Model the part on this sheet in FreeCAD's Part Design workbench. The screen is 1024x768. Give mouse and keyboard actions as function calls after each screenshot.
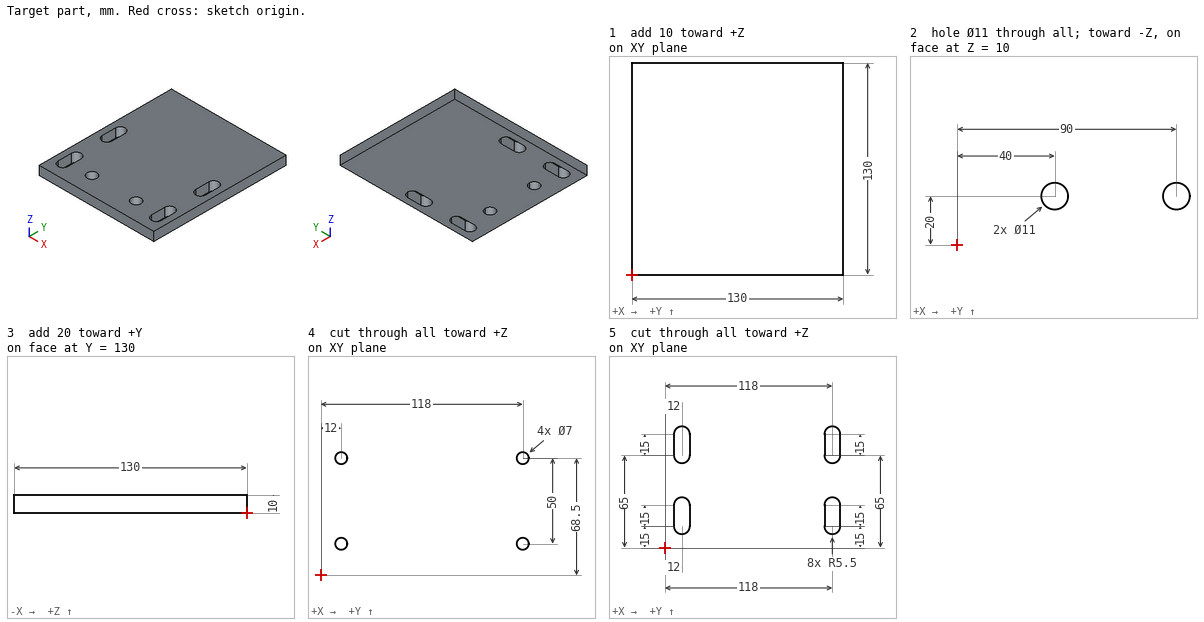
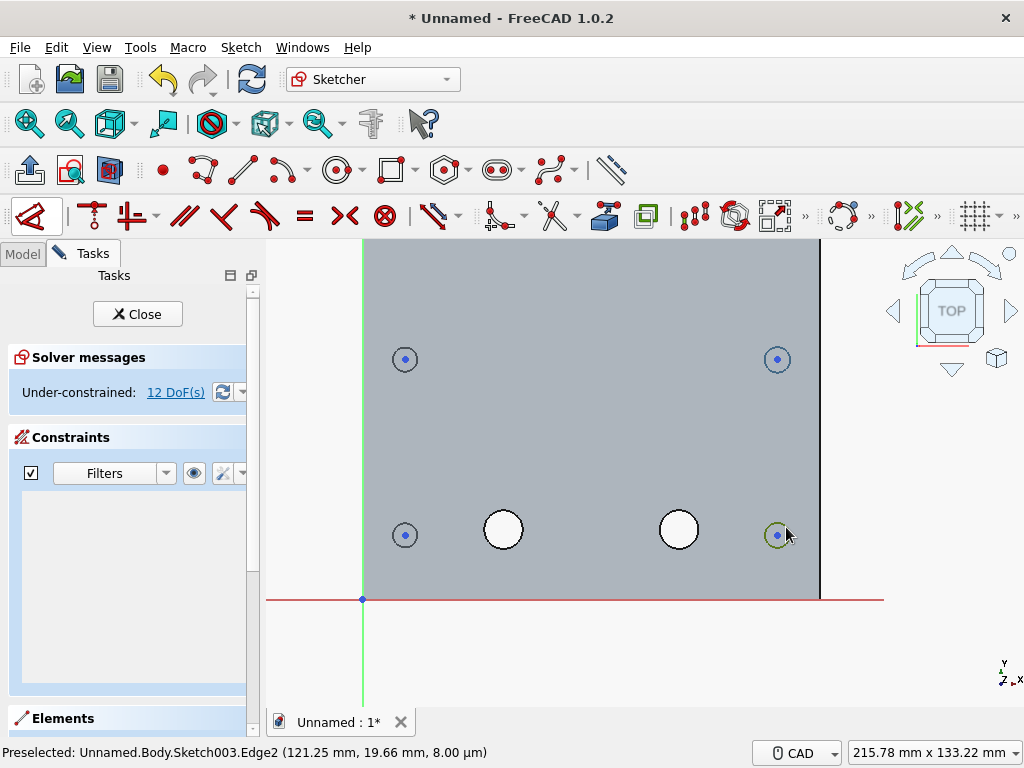
click(414, 351)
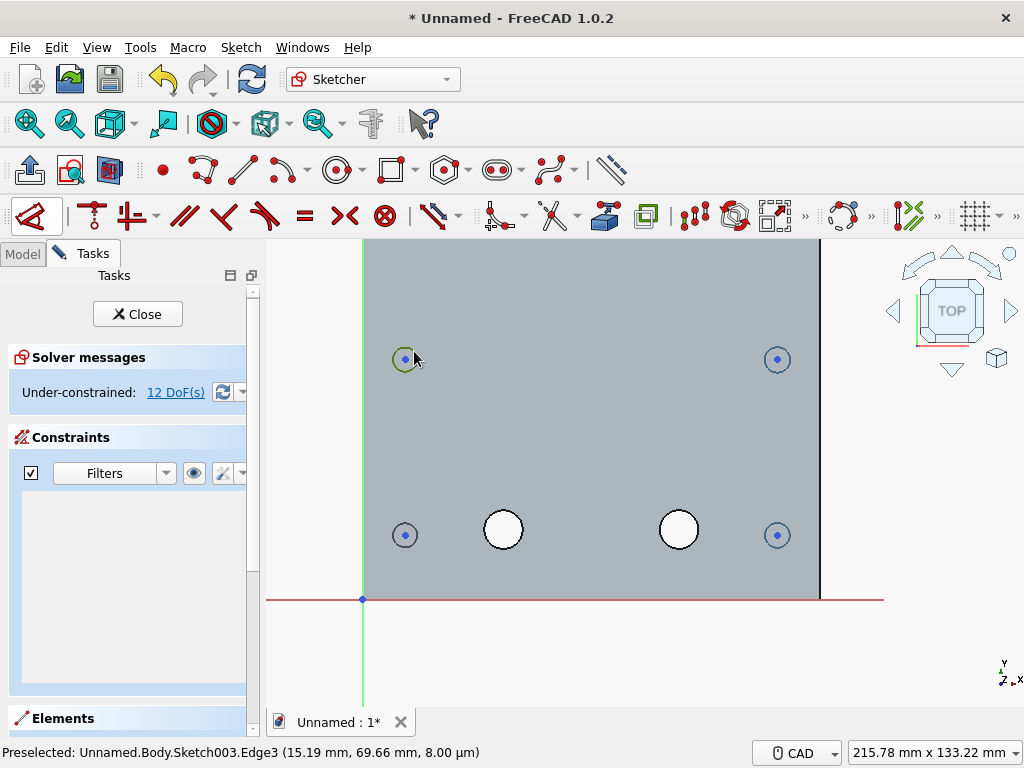
click(414, 527)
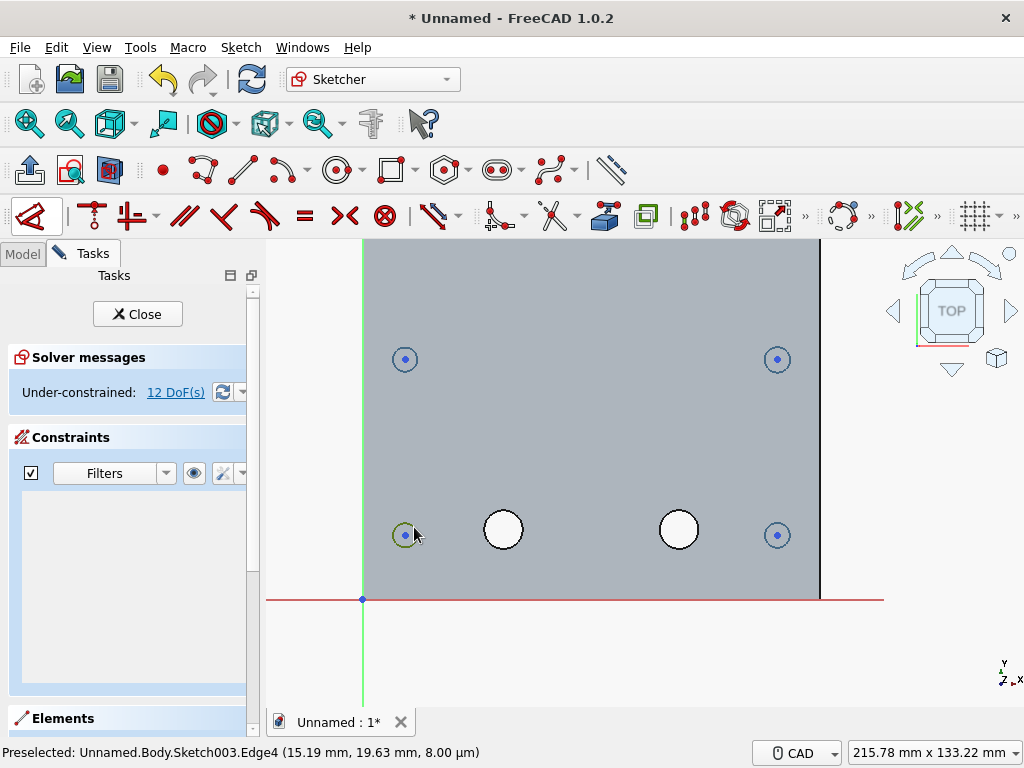
click(306, 216)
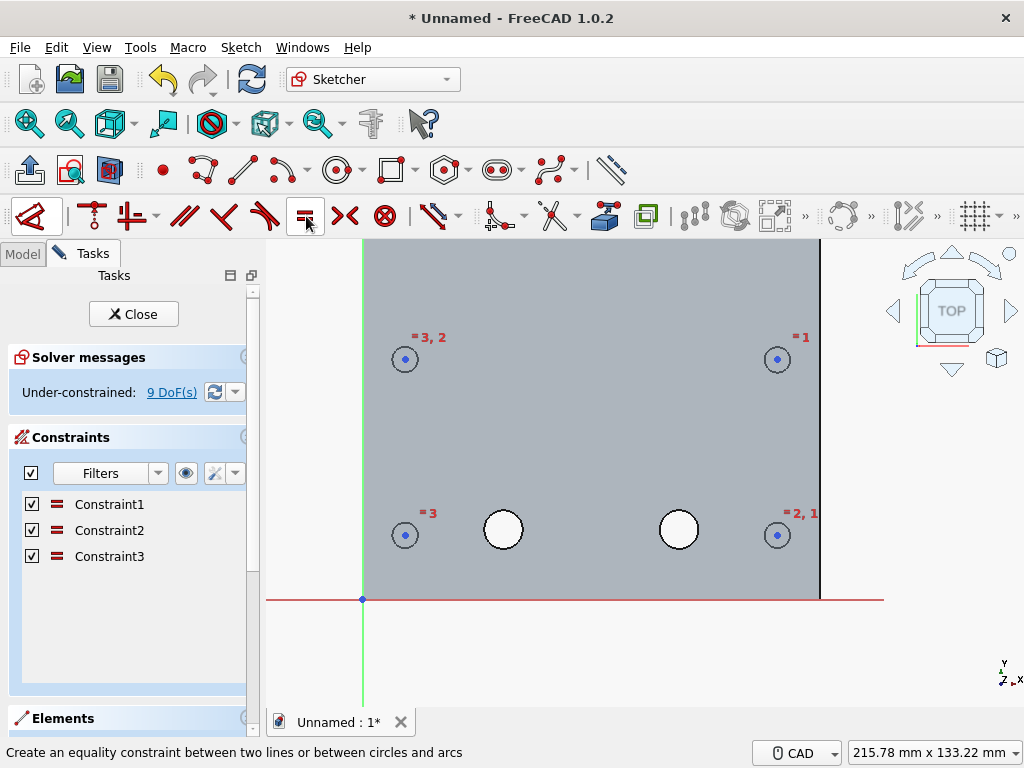
click(777, 360)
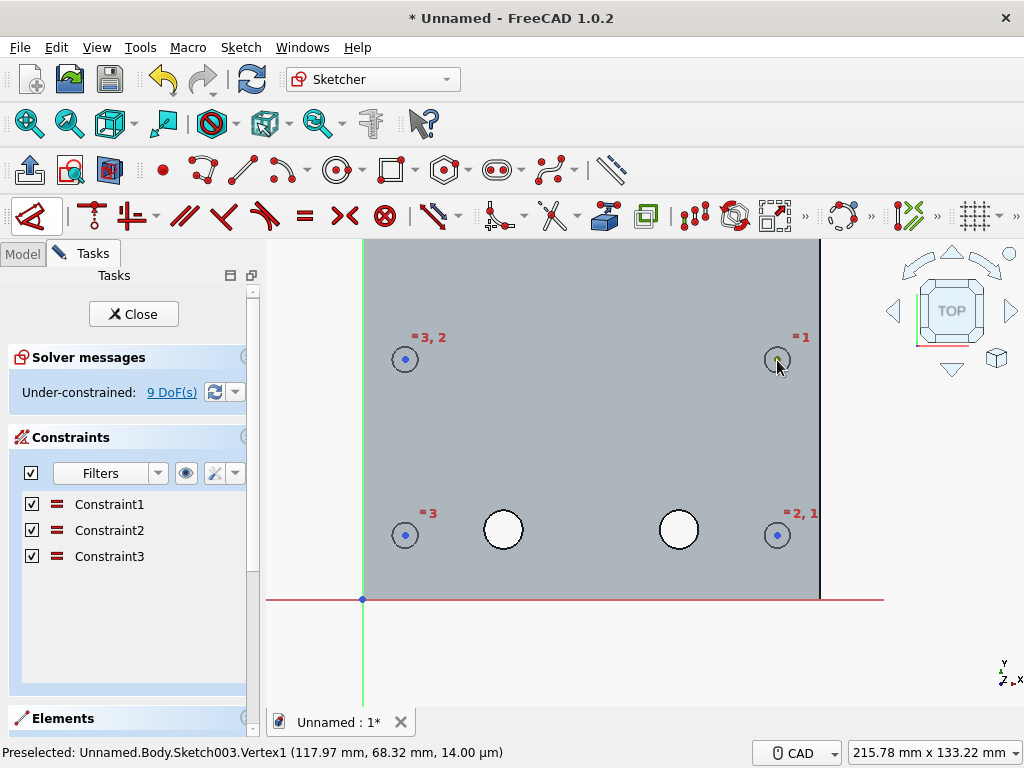
click(777, 535)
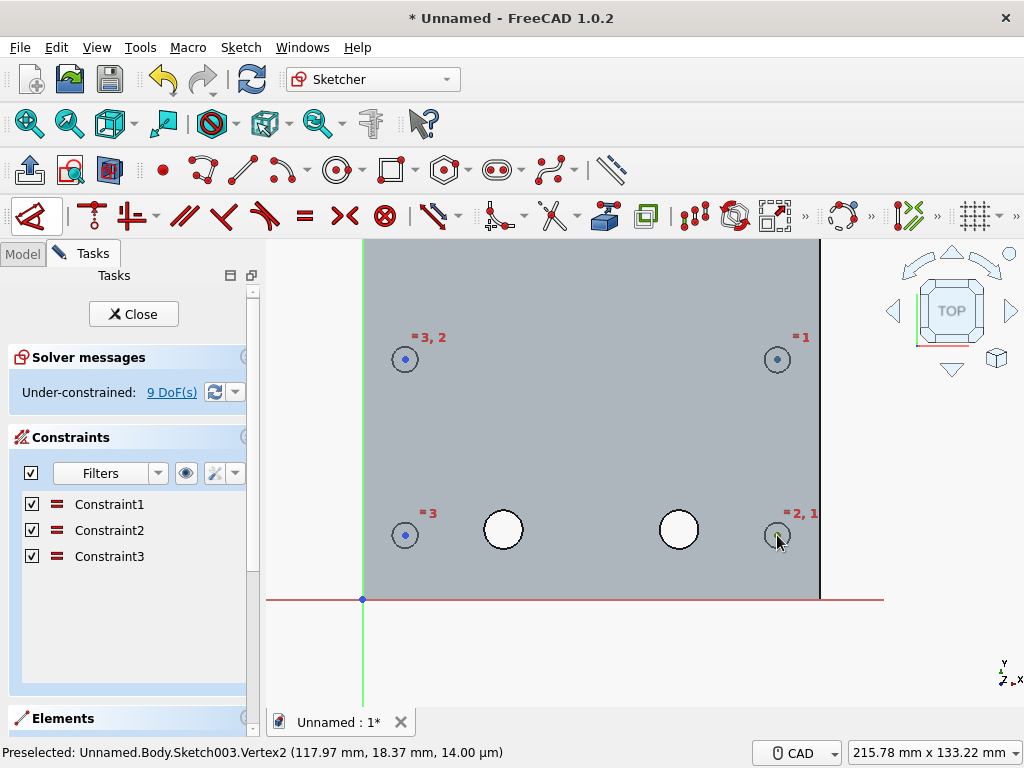
key(v)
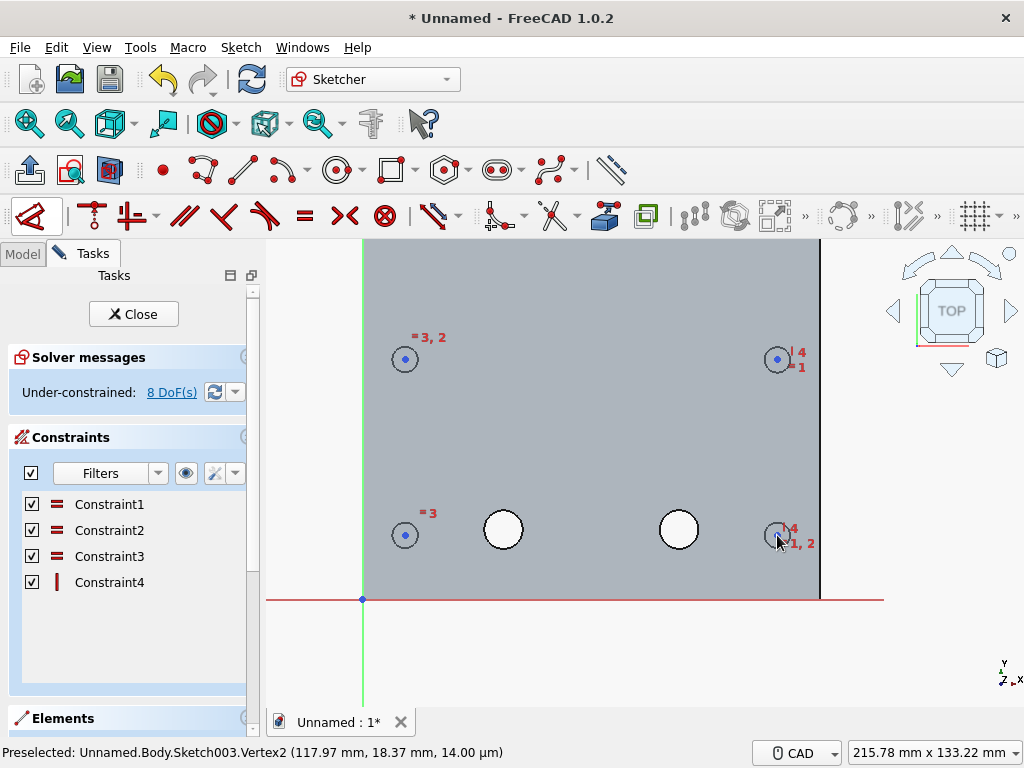
click(777, 360)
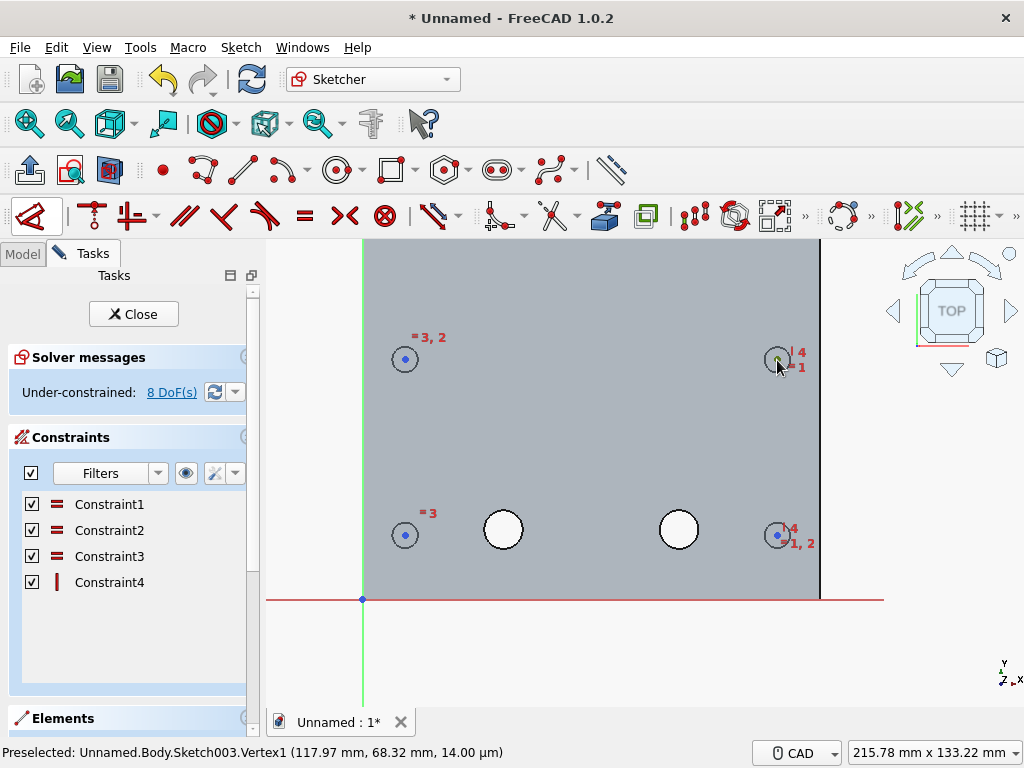
click(405, 360)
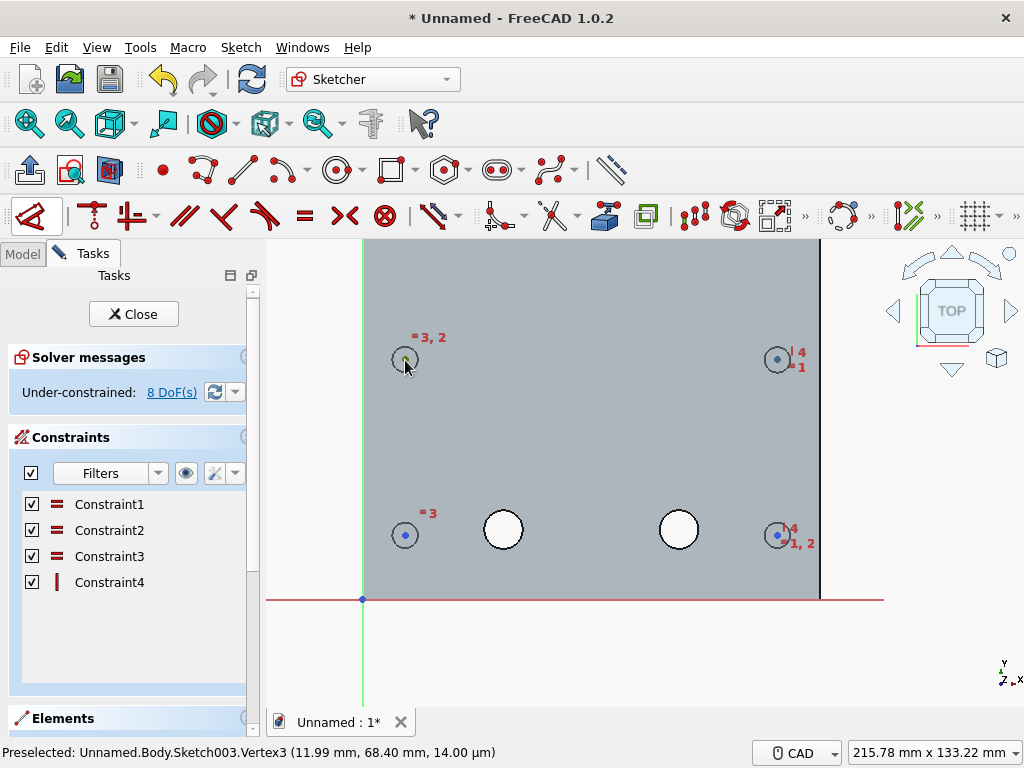
click(158, 216)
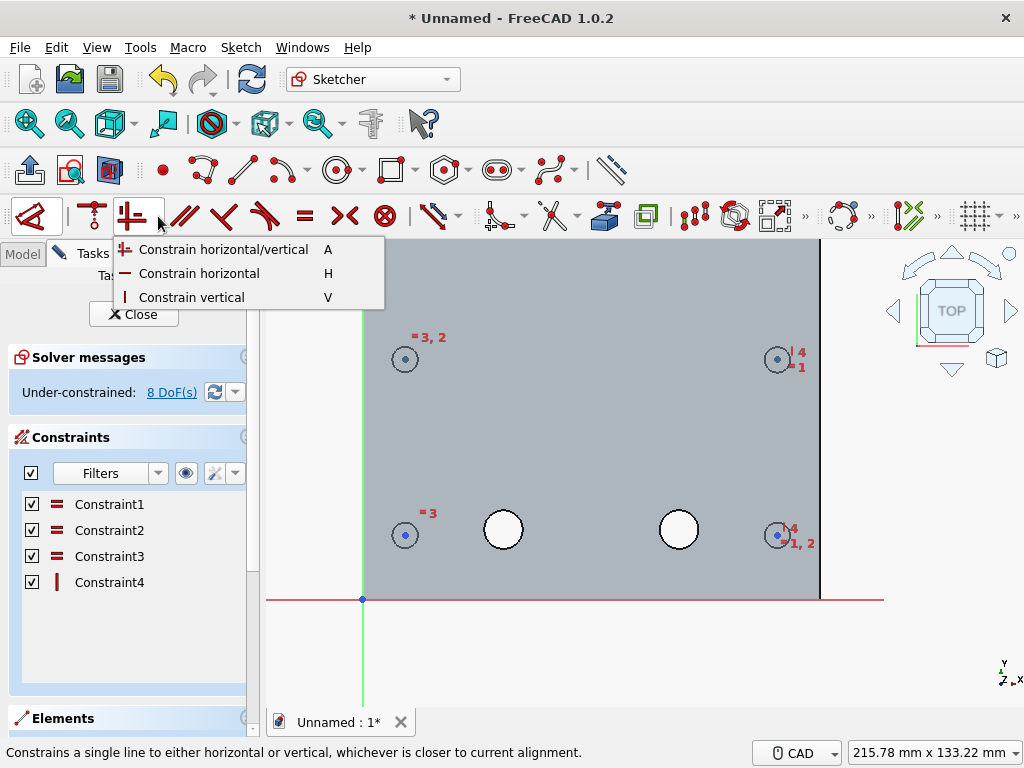
click(249, 273)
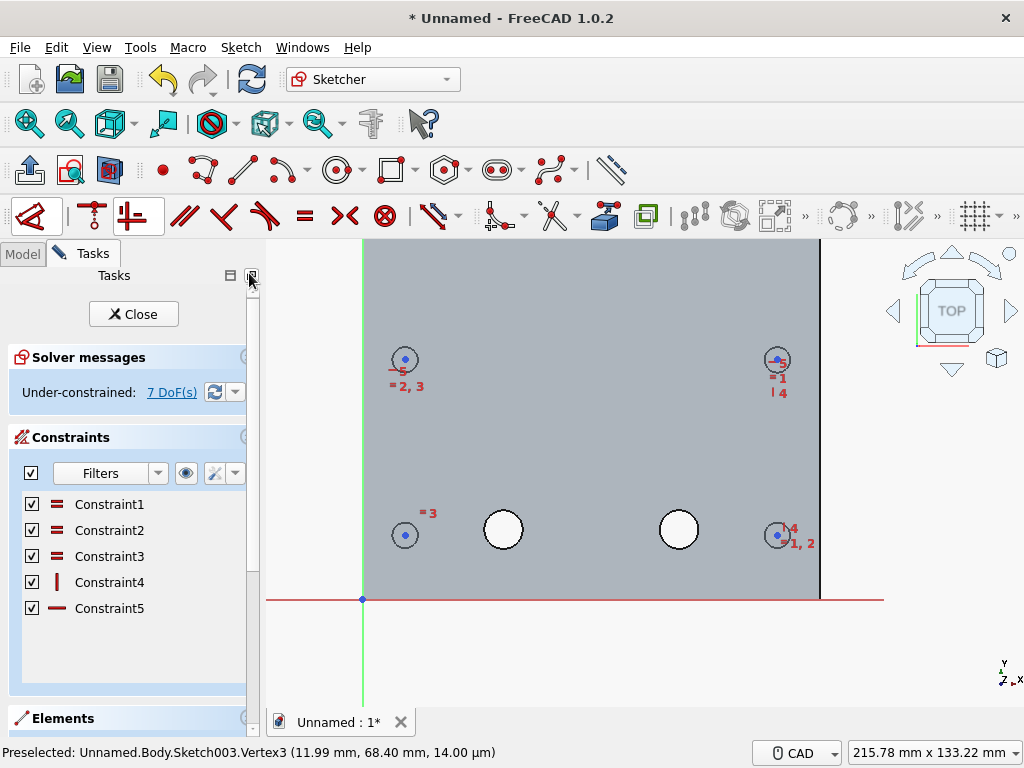
click(405, 360)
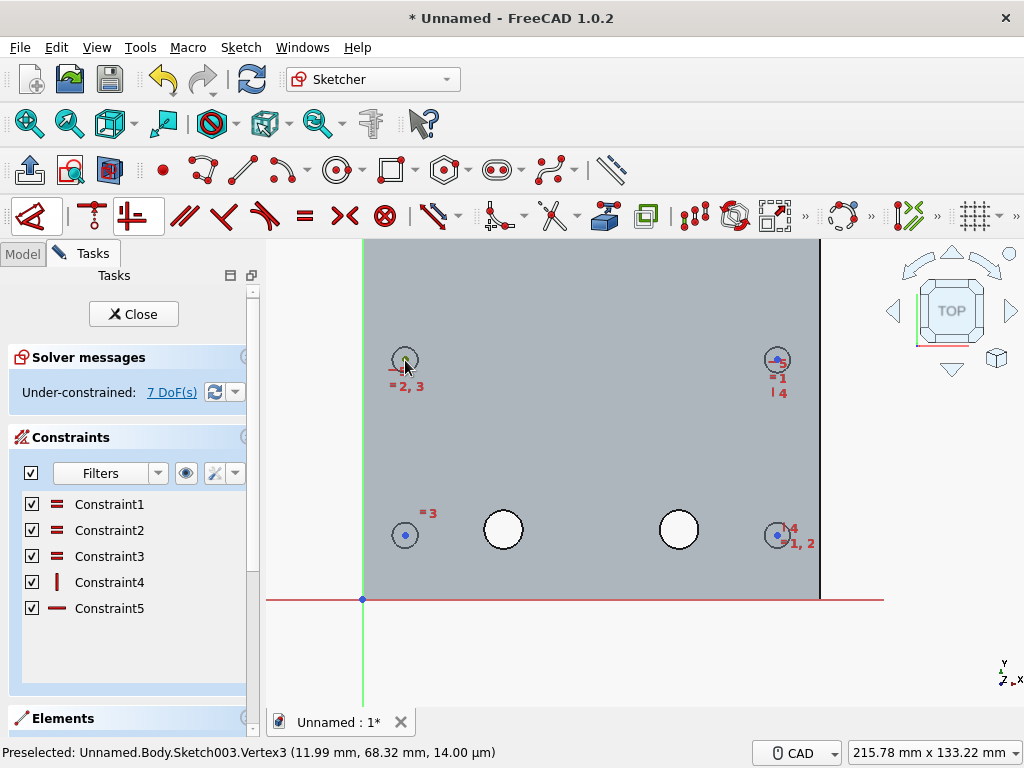
click(405, 535)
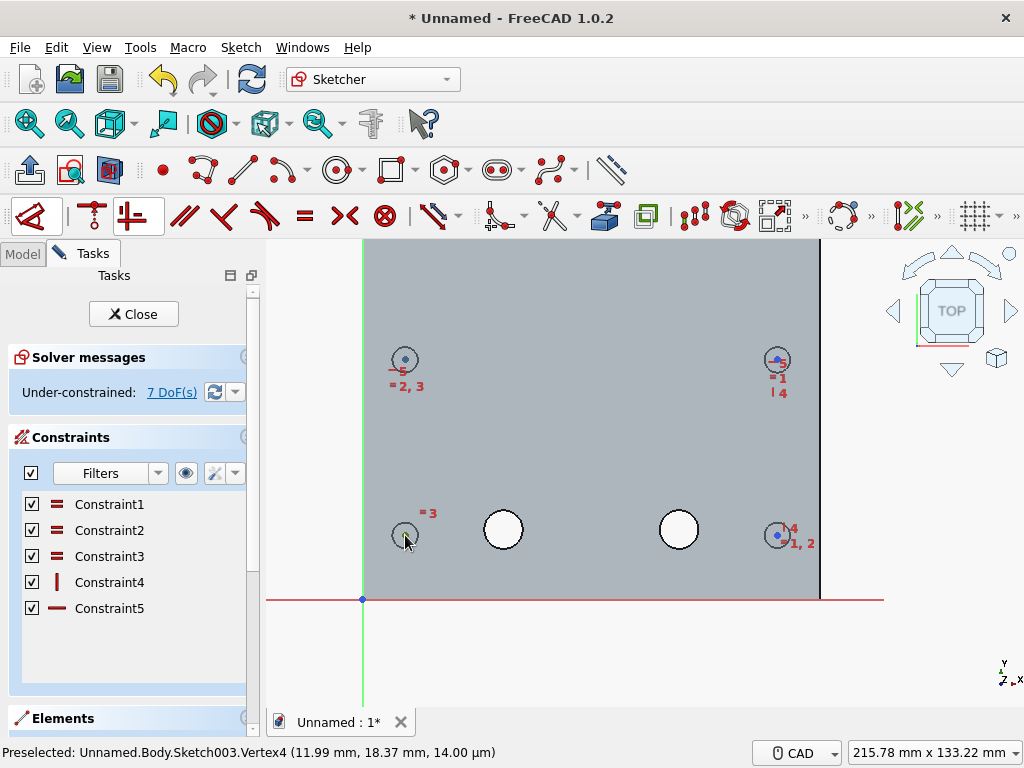
click(158, 216)